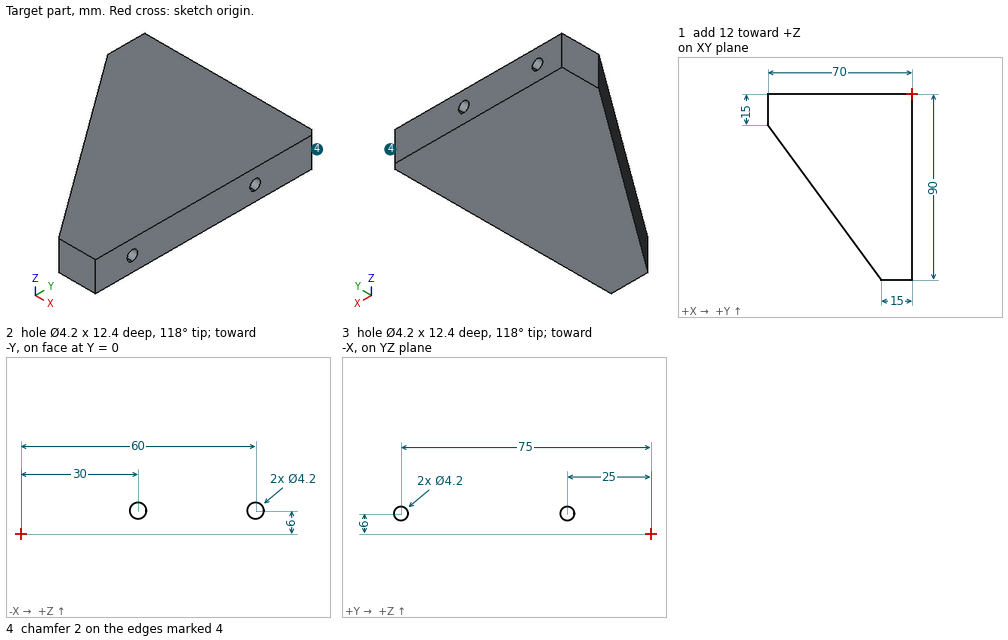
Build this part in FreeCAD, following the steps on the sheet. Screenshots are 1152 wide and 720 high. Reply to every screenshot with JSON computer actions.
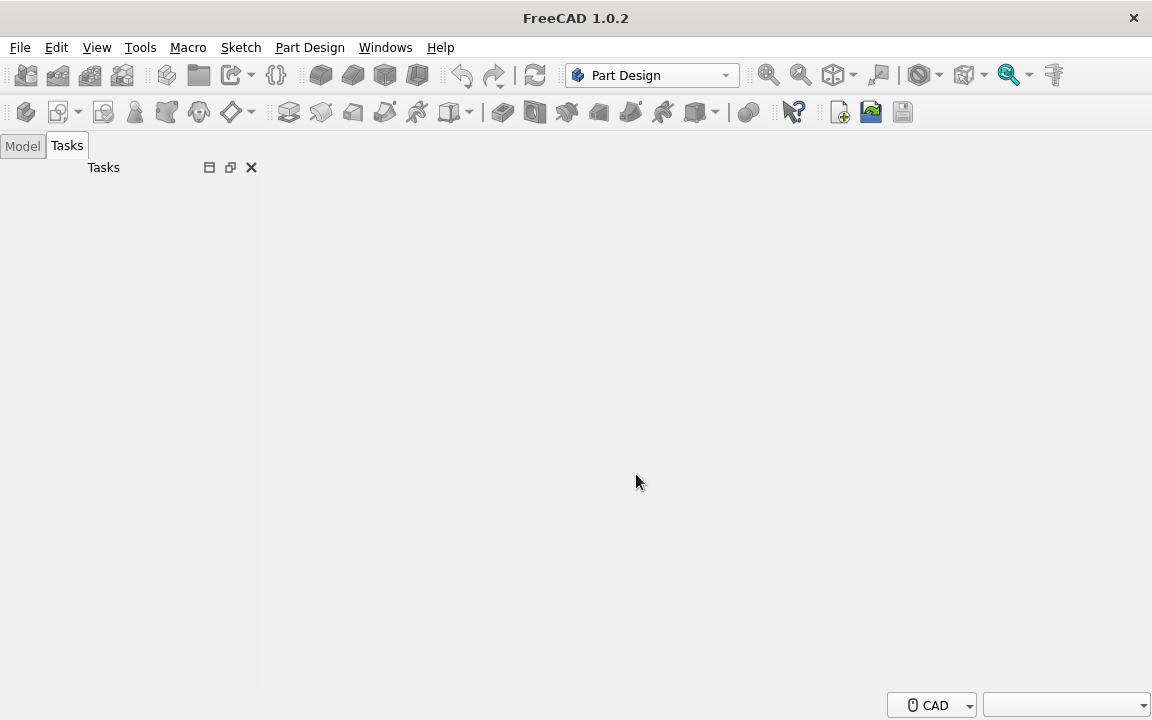
{"action": "left_click", "coordinate": [840, 112]}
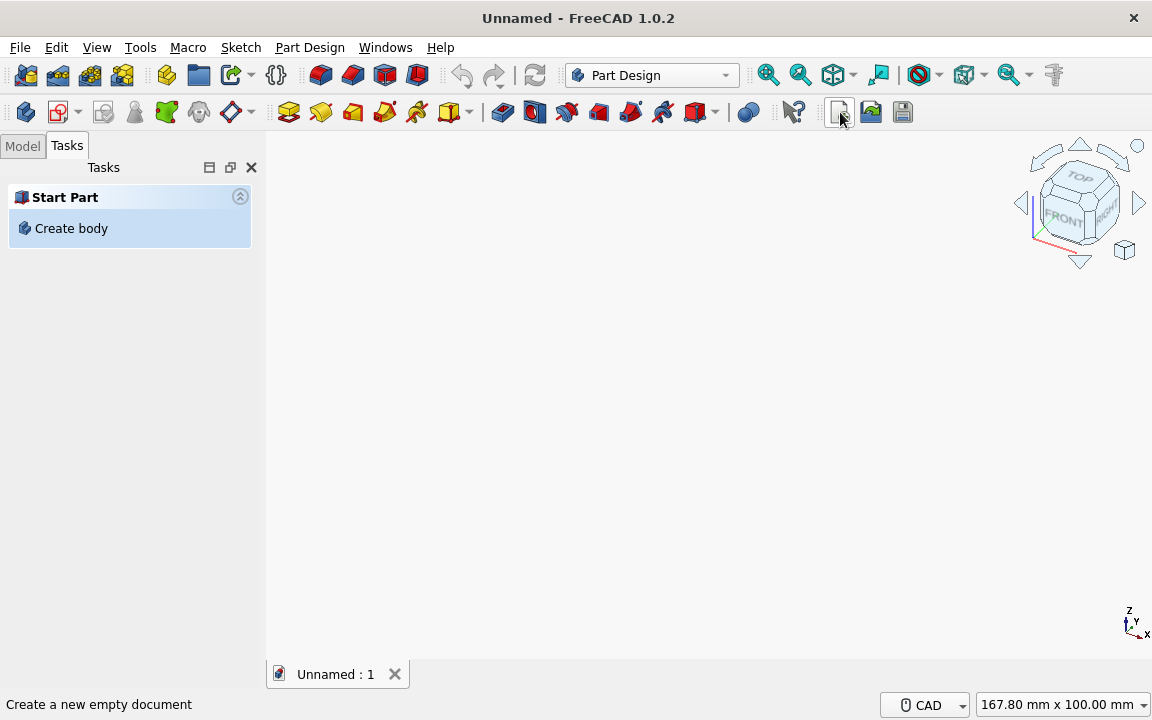
{"action": "left_click", "coordinate": [58, 112]}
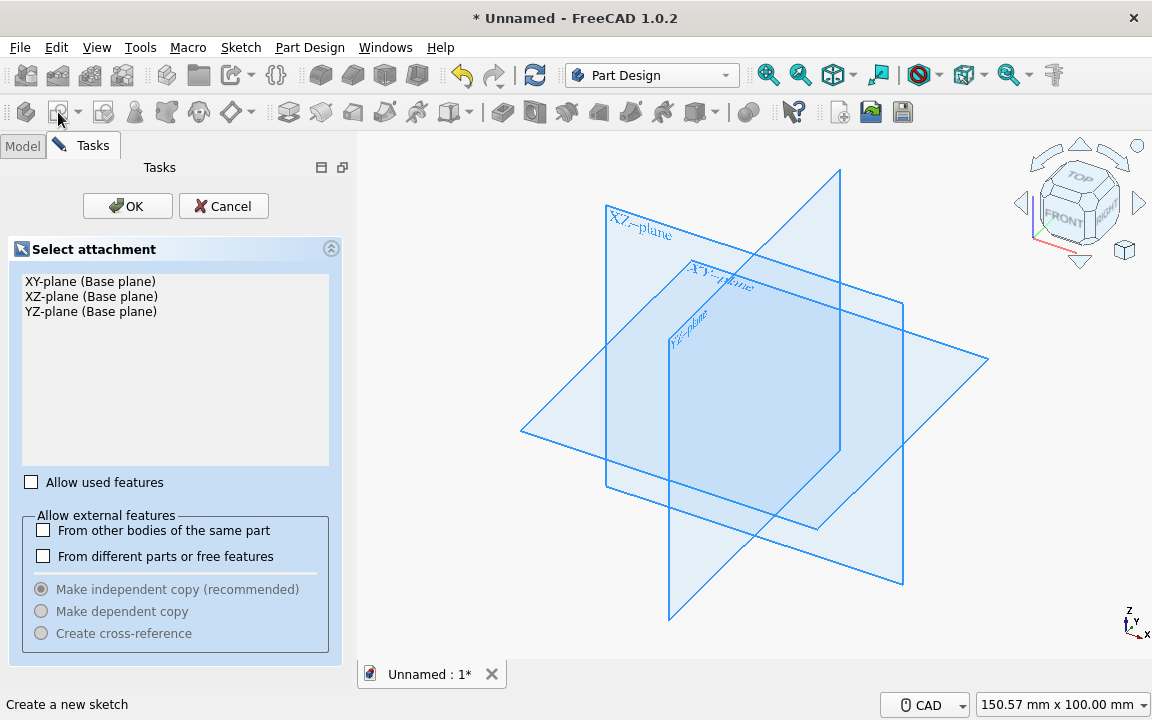
{"action": "left_click", "coordinate": [82, 282]}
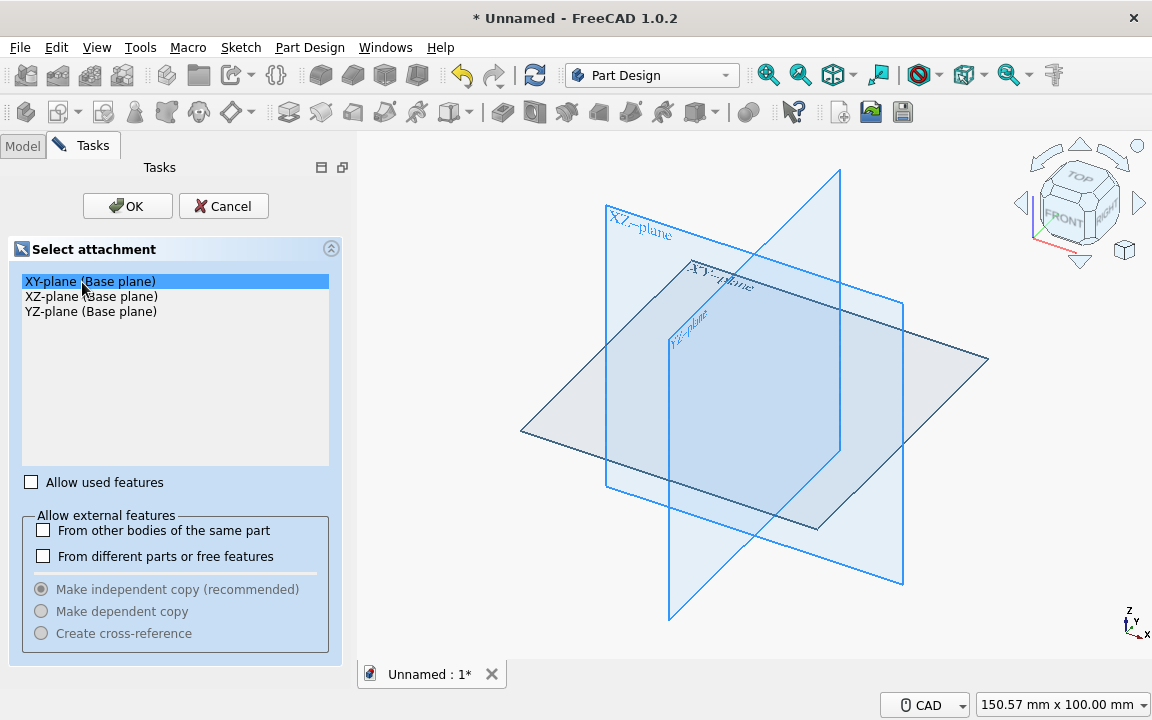
{"action": "left_click", "coordinate": [128, 206]}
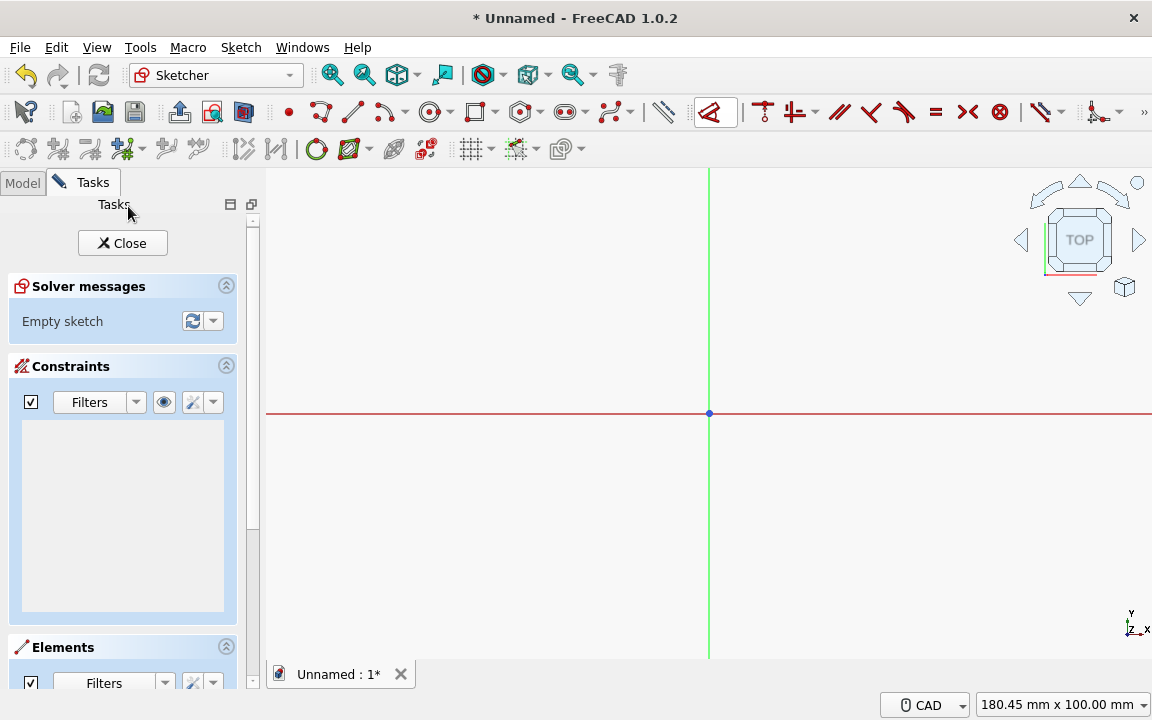
{"action": "scroll", "coordinate": [766, 196], "scroll_direction": "down", "scroll_amount": 3}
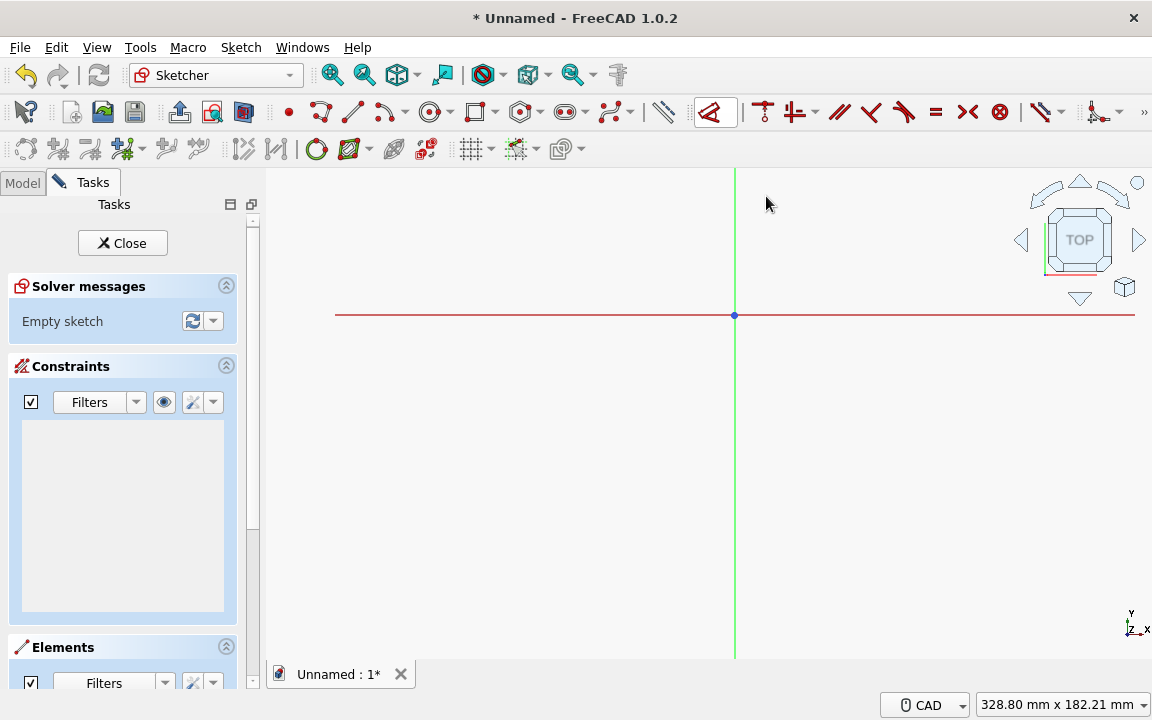
{"action": "left_click", "coordinate": [322, 112]}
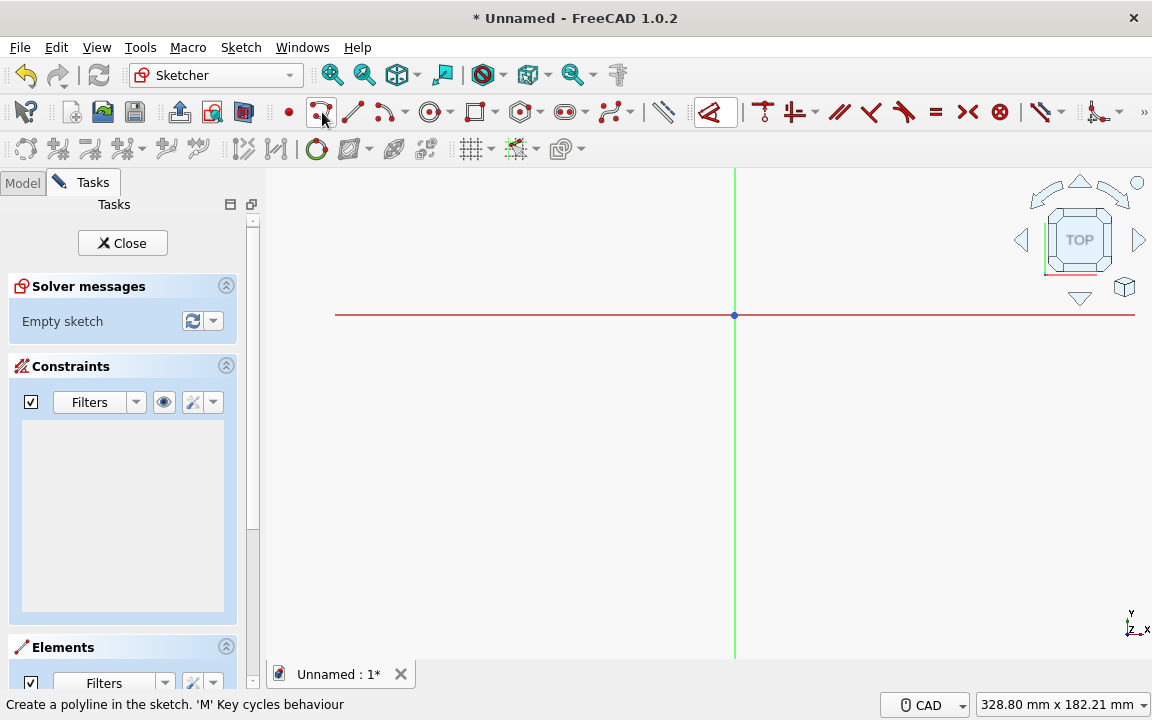
{"action": "left_click", "coordinate": [735, 315]}
{"action": "left_click", "coordinate": [546, 324]}
{"action": "left_click", "coordinate": [546, 356]}
{"action": "left_click", "coordinate": [695, 558]}
{"action": "left_click", "coordinate": [726, 558]}
{"action": "left_click", "coordinate": [735, 315]}
{"action": "key", "text": "Escape"}
{"action": "key", "text": "Escape"}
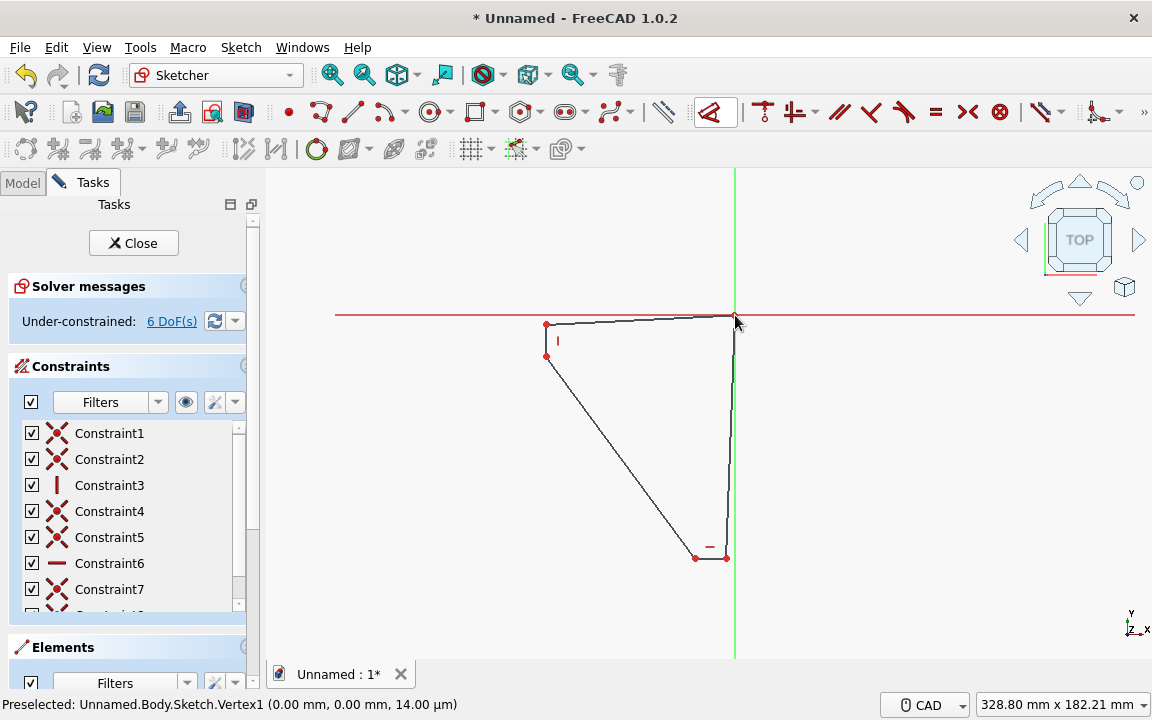
{"action": "left_click", "coordinate": [678, 318]}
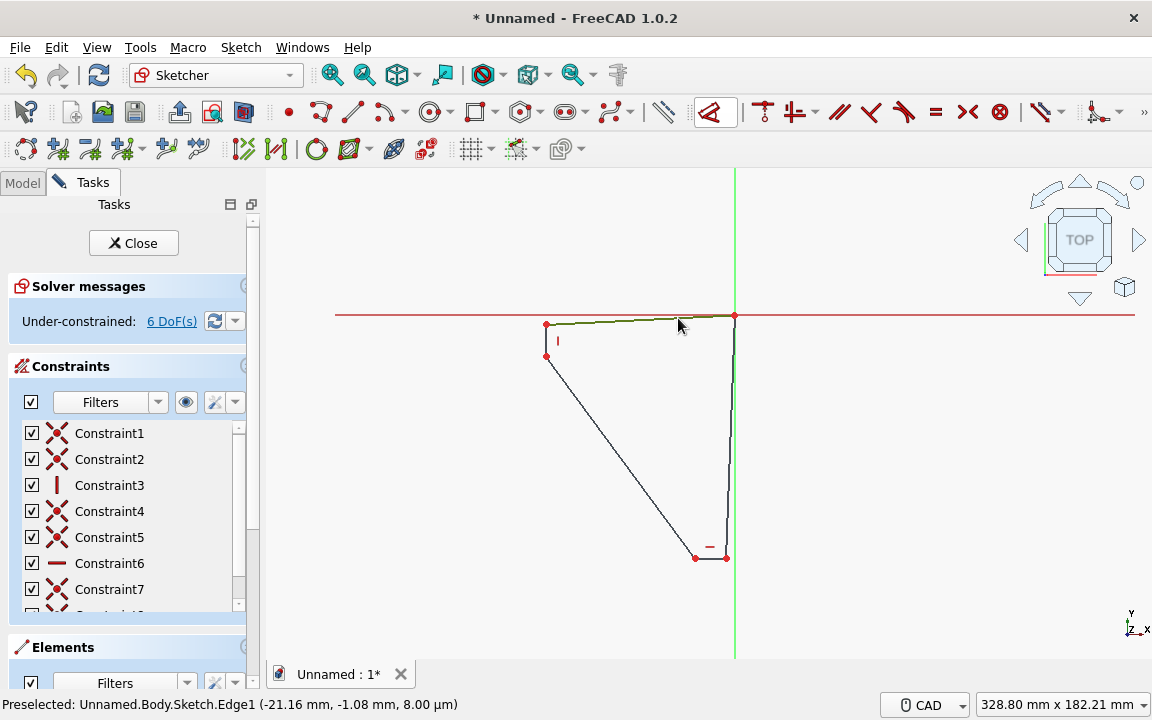
{"action": "key", "text": "h"}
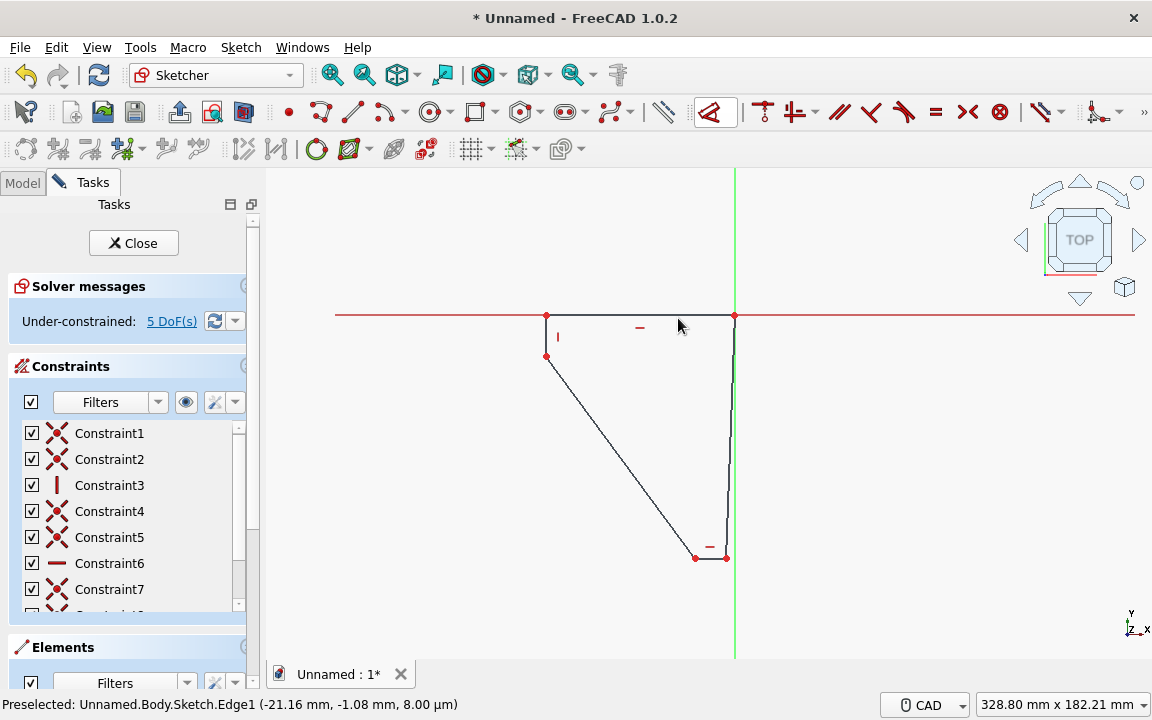
{"action": "left_click", "coordinate": [732, 388]}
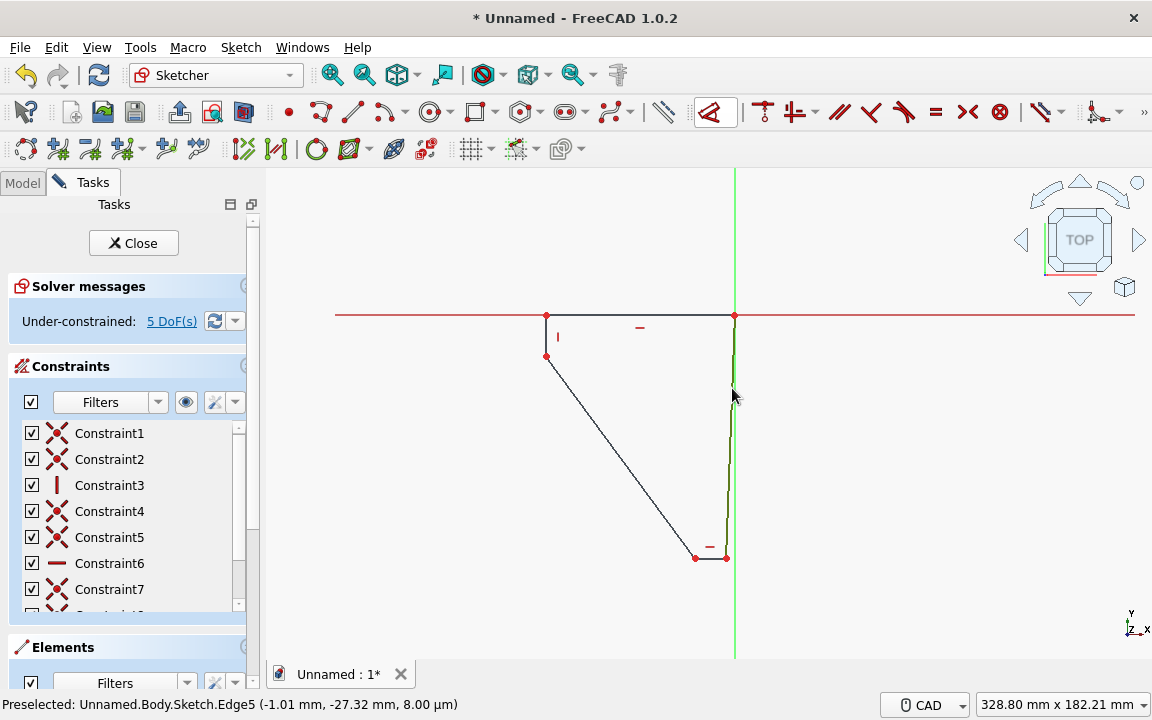
{"action": "left_click", "coordinate": [818, 112]}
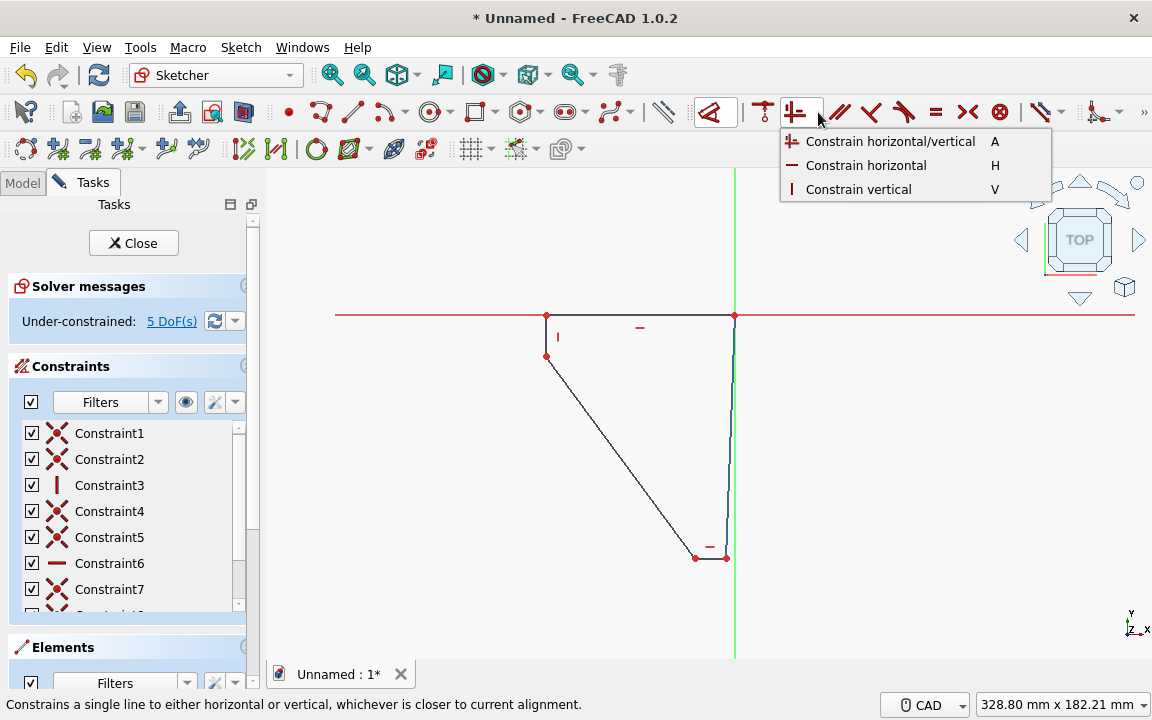
{"action": "left_click", "coordinate": [916, 189]}